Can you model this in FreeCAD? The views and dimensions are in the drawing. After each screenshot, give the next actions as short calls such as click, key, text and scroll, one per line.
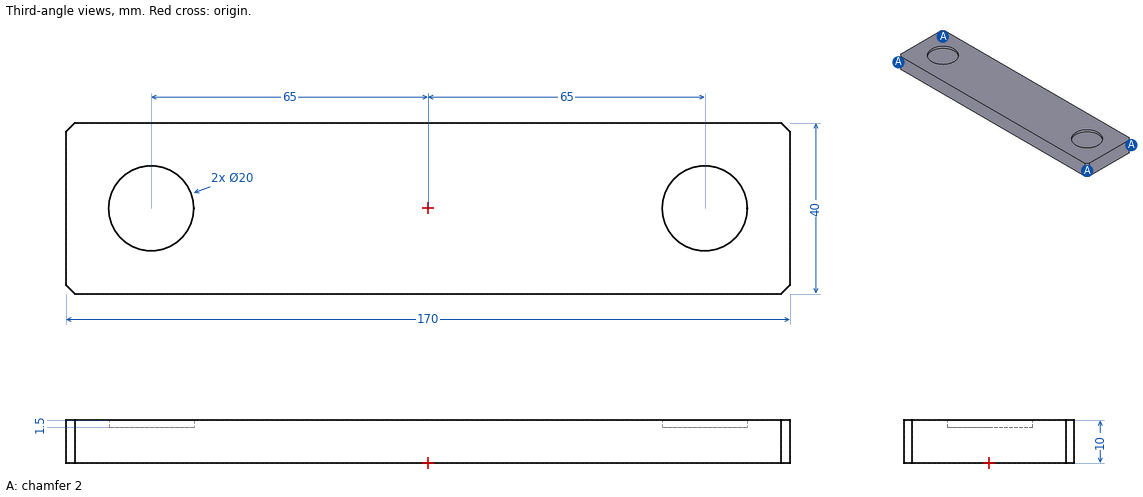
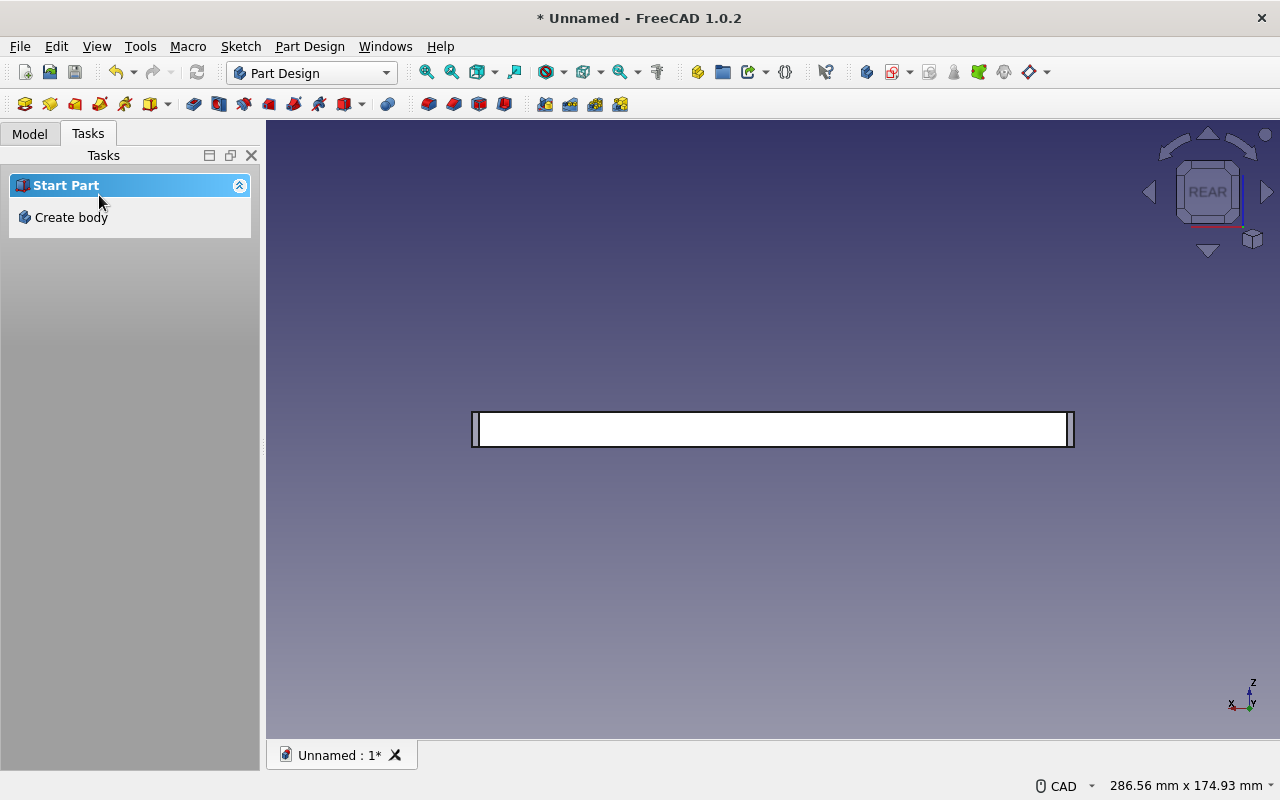
key(0)